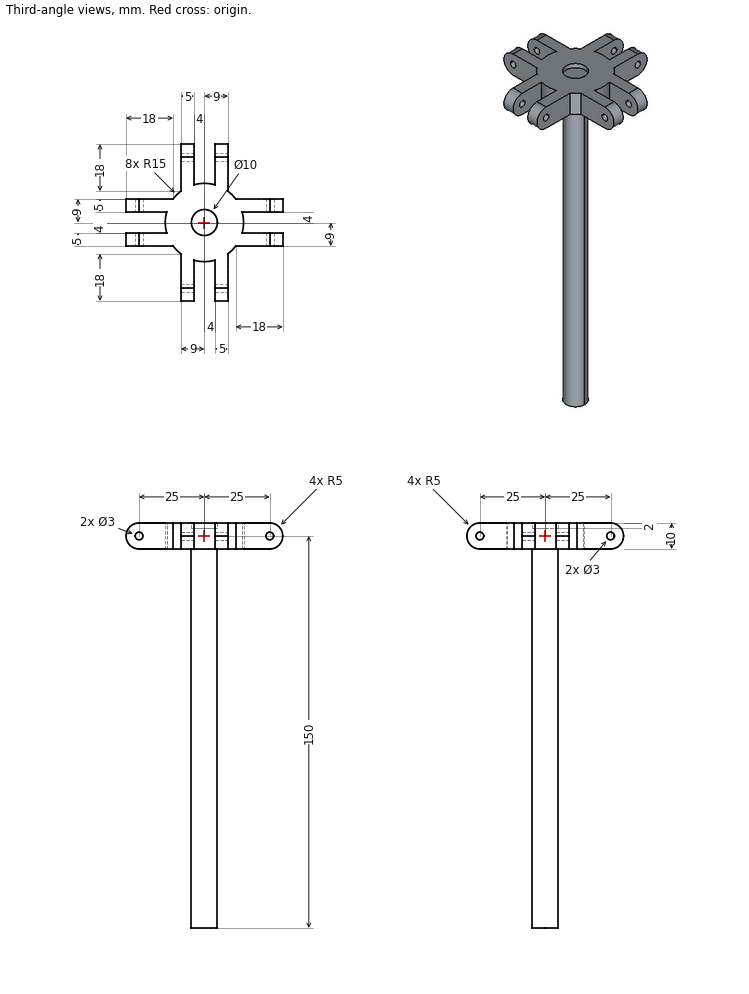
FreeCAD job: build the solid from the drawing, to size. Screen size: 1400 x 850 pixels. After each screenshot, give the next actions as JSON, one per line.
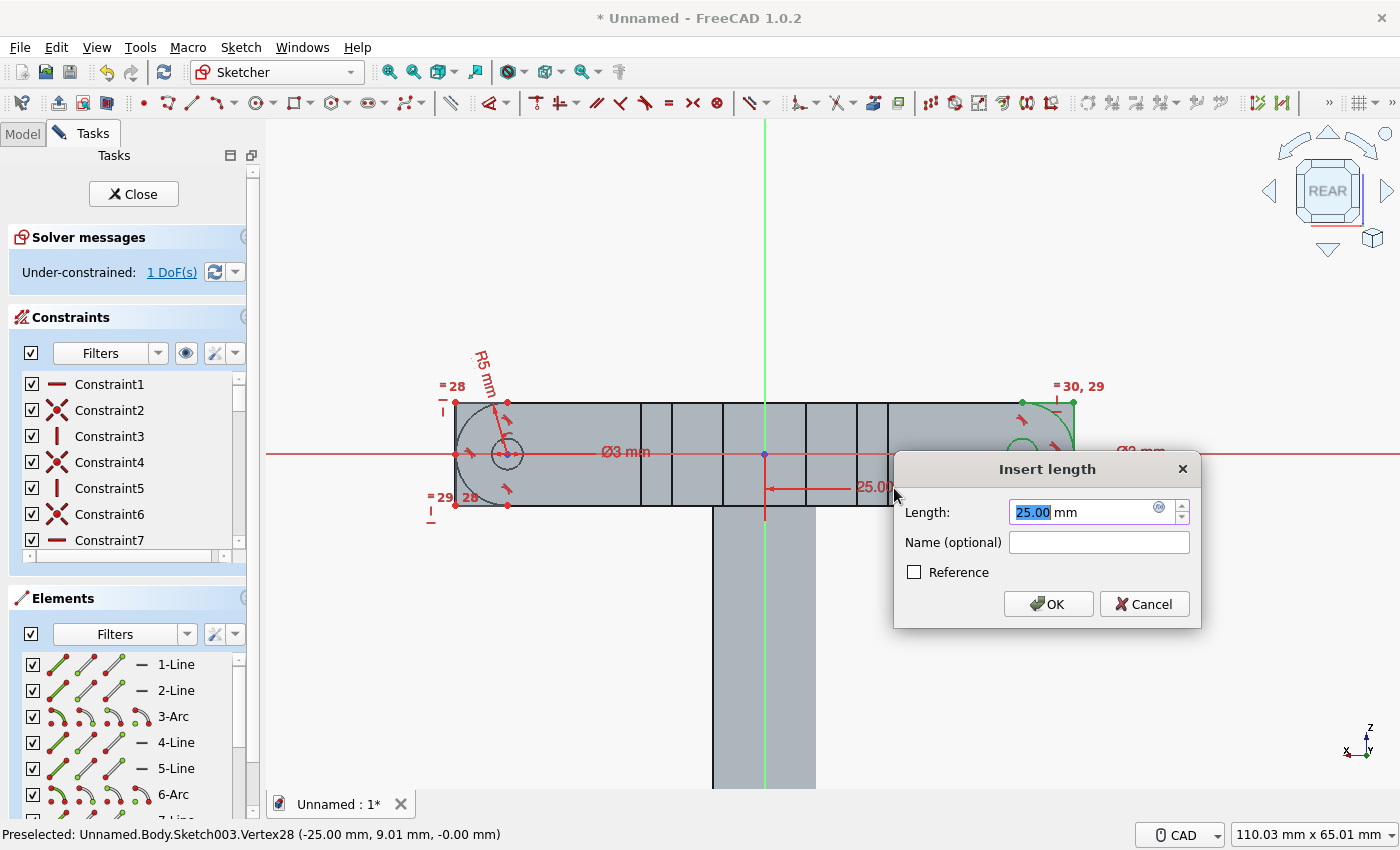
{"action": "type", "text": "25"}
{"action": "key", "text": "Return"}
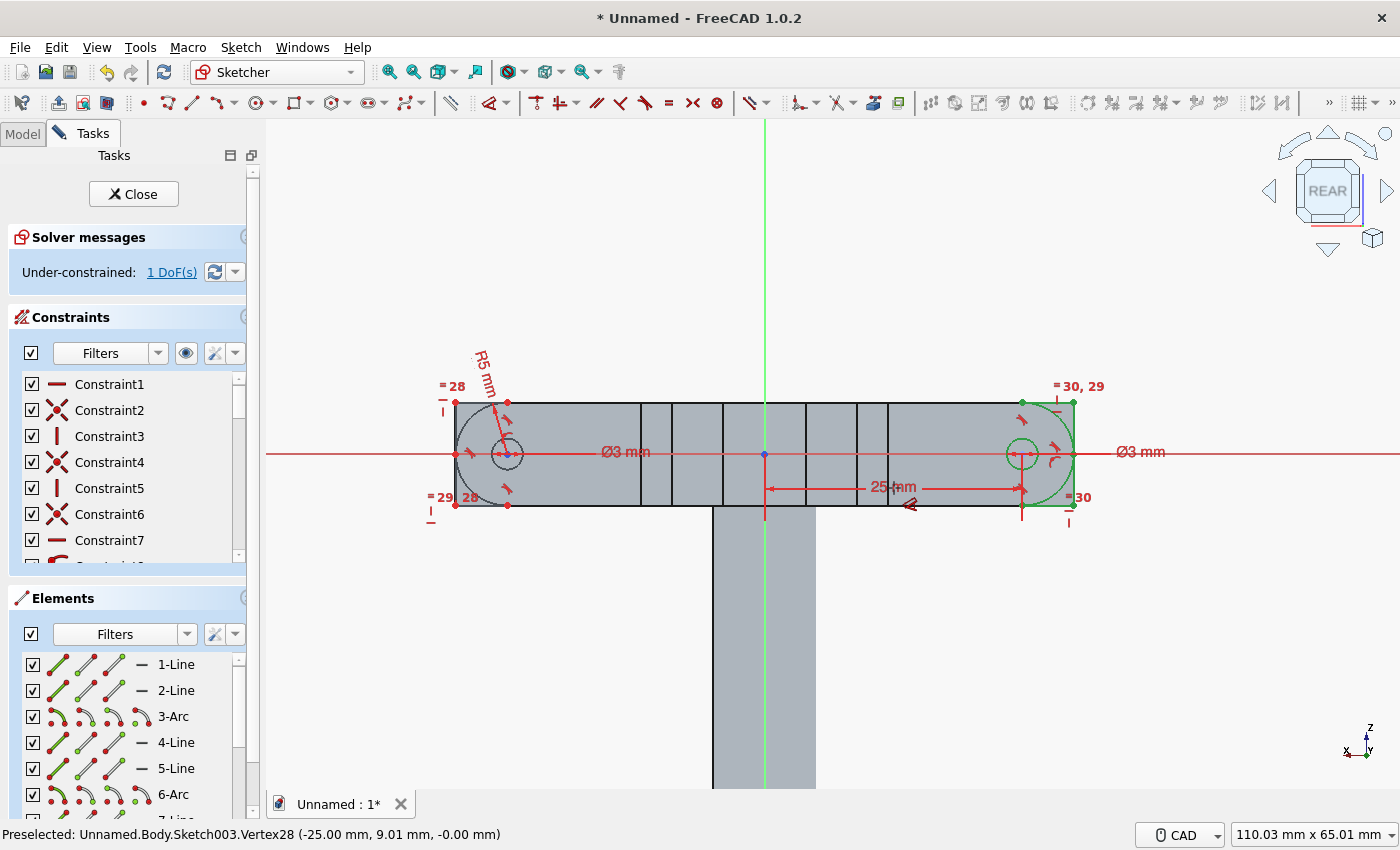
{"action": "left_click", "coordinate": [507, 454]}
{"action": "left_click", "coordinate": [636, 488]}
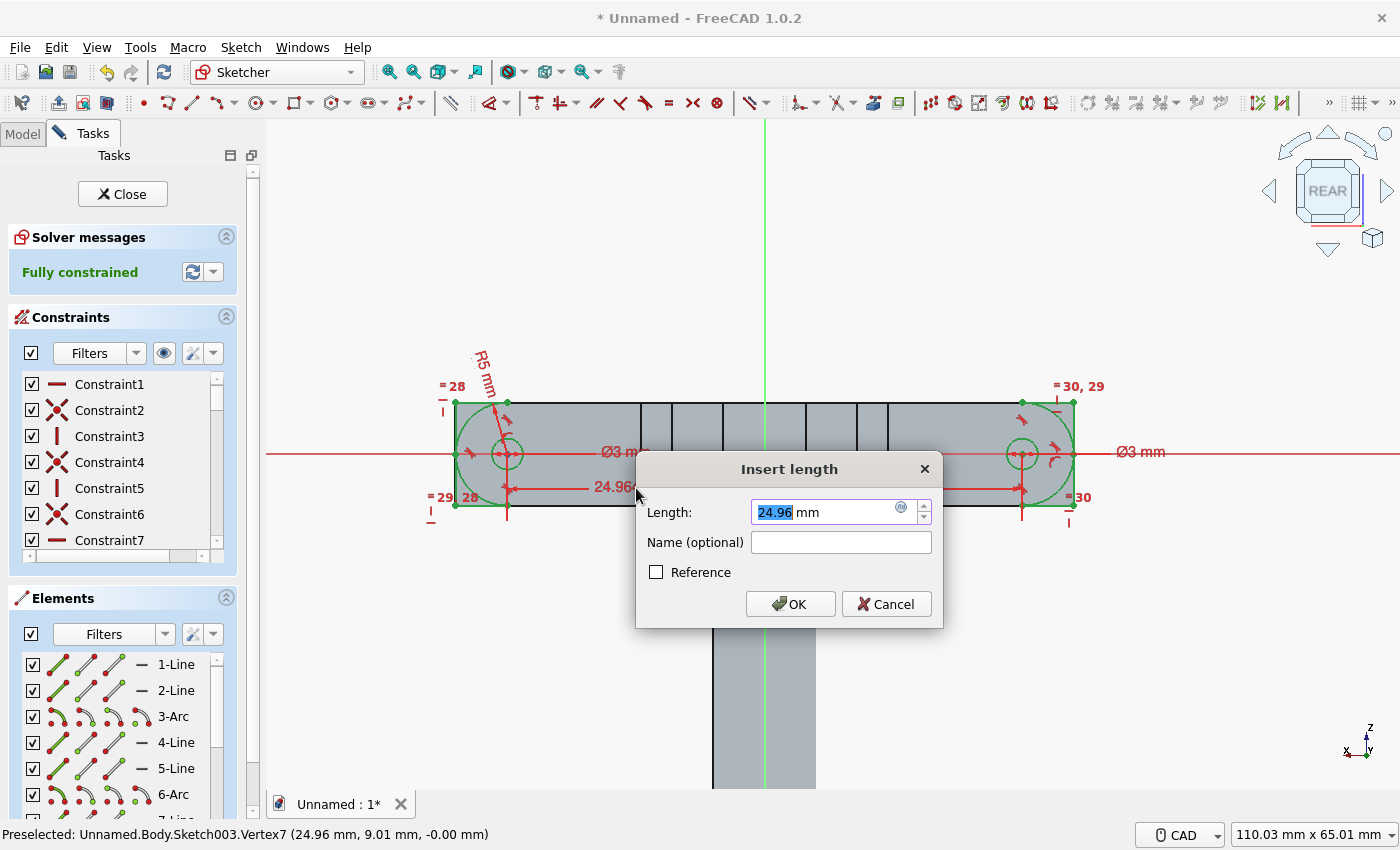
{"action": "type", "text": "25"}
{"action": "key", "text": "Return"}
{"action": "key", "text": "Escape"}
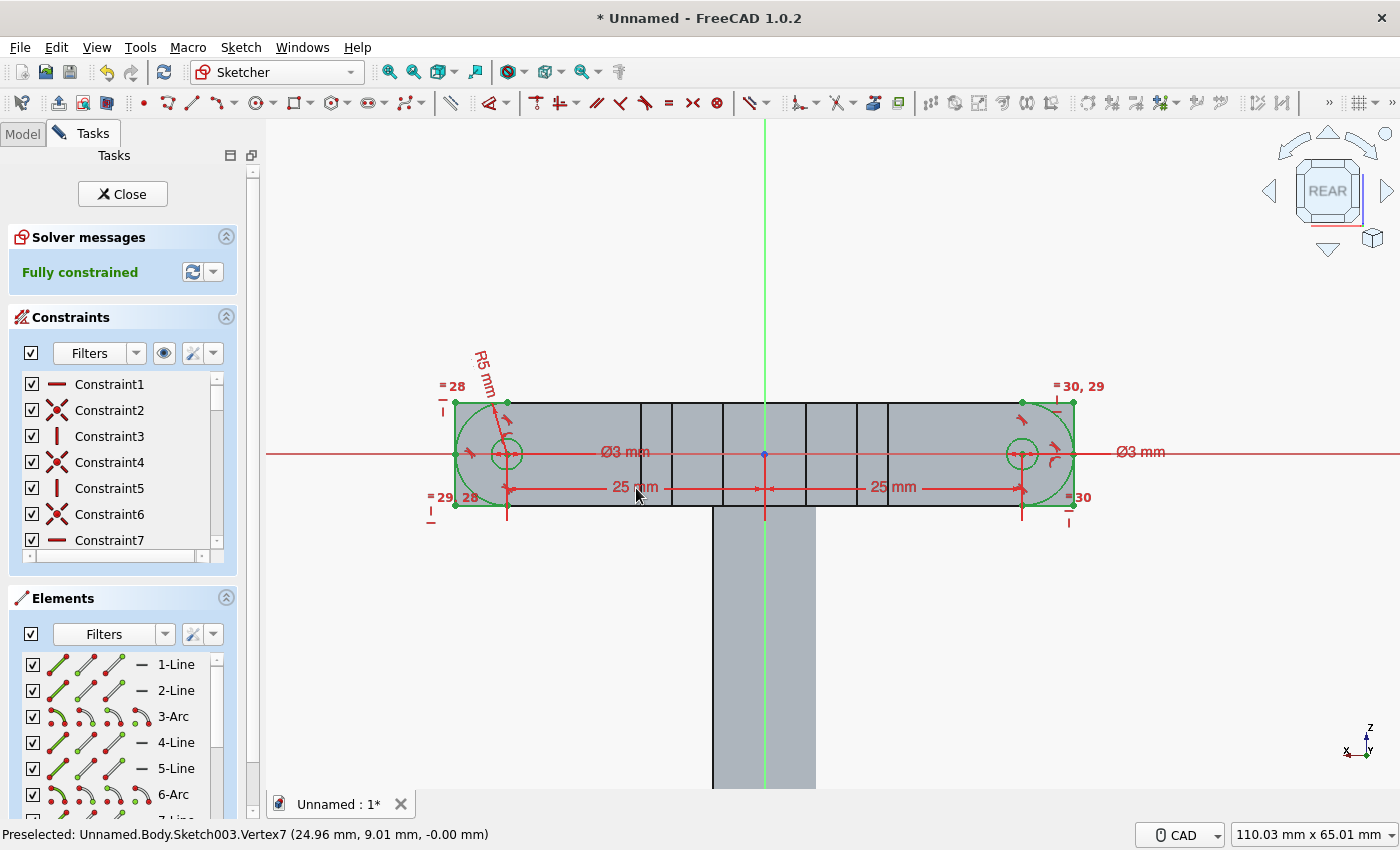
{"action": "left_click", "coordinate": [123, 194]}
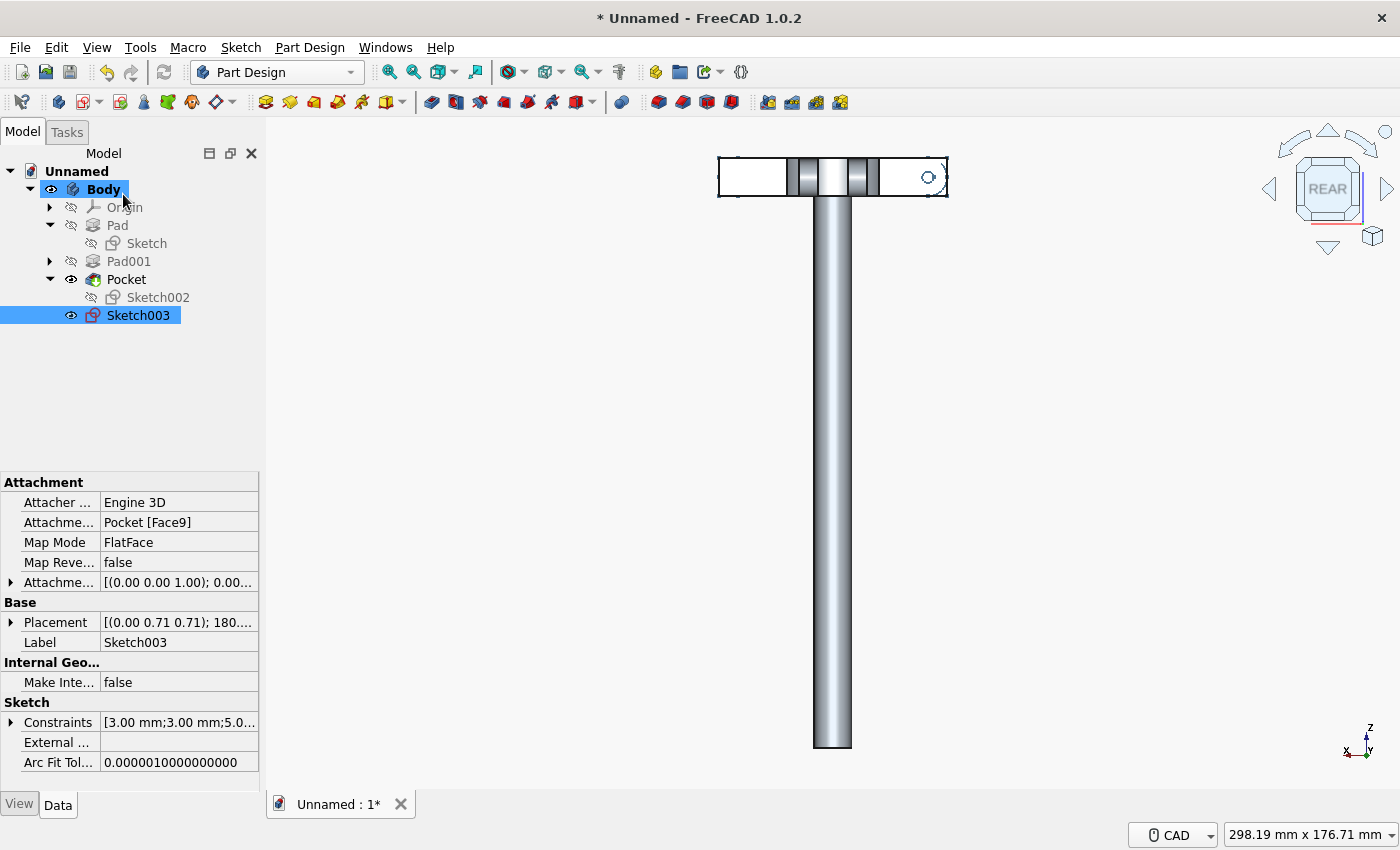
{"action": "left_click", "coordinate": [432, 102]}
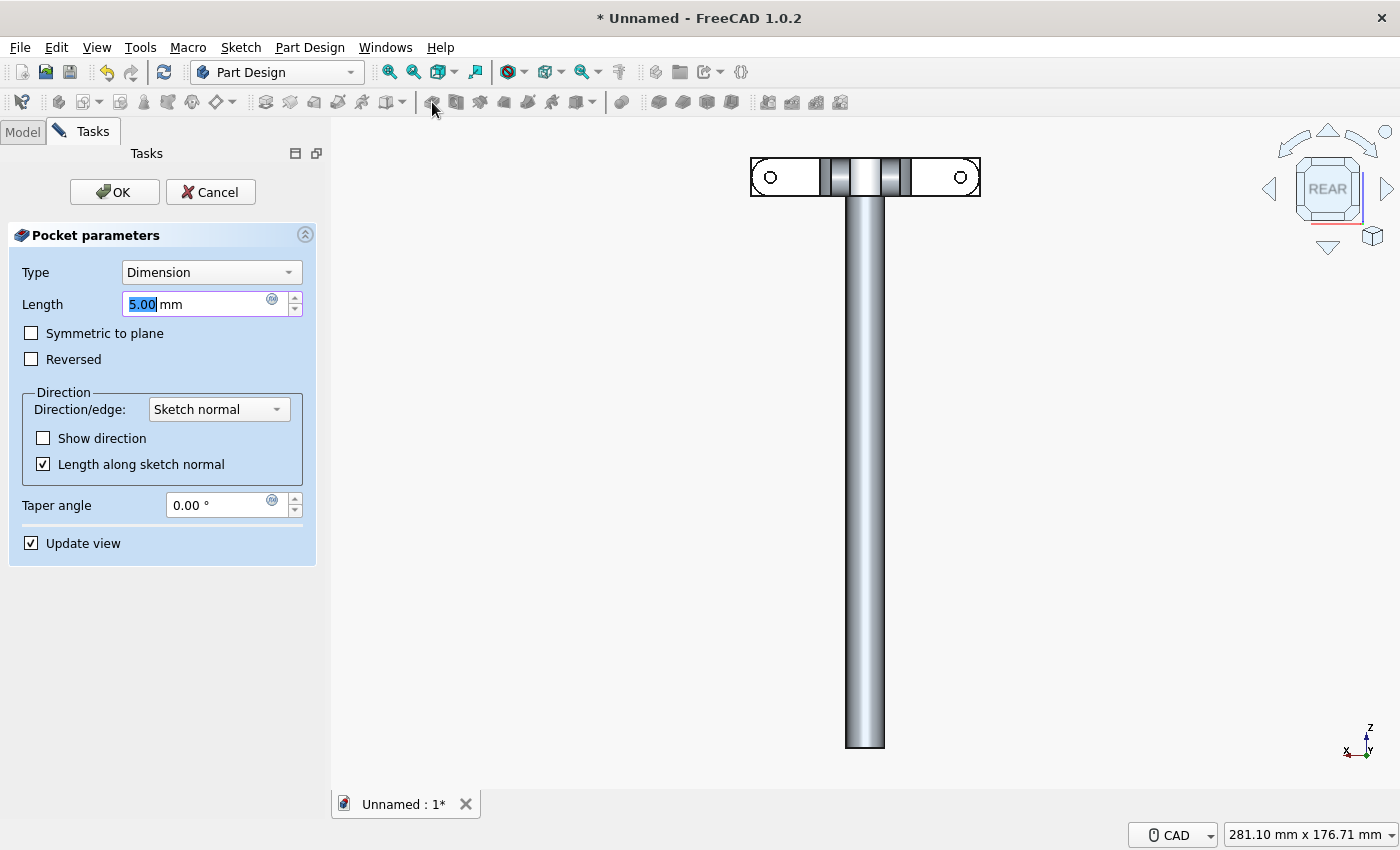
{"action": "left_click", "coordinate": [212, 272]}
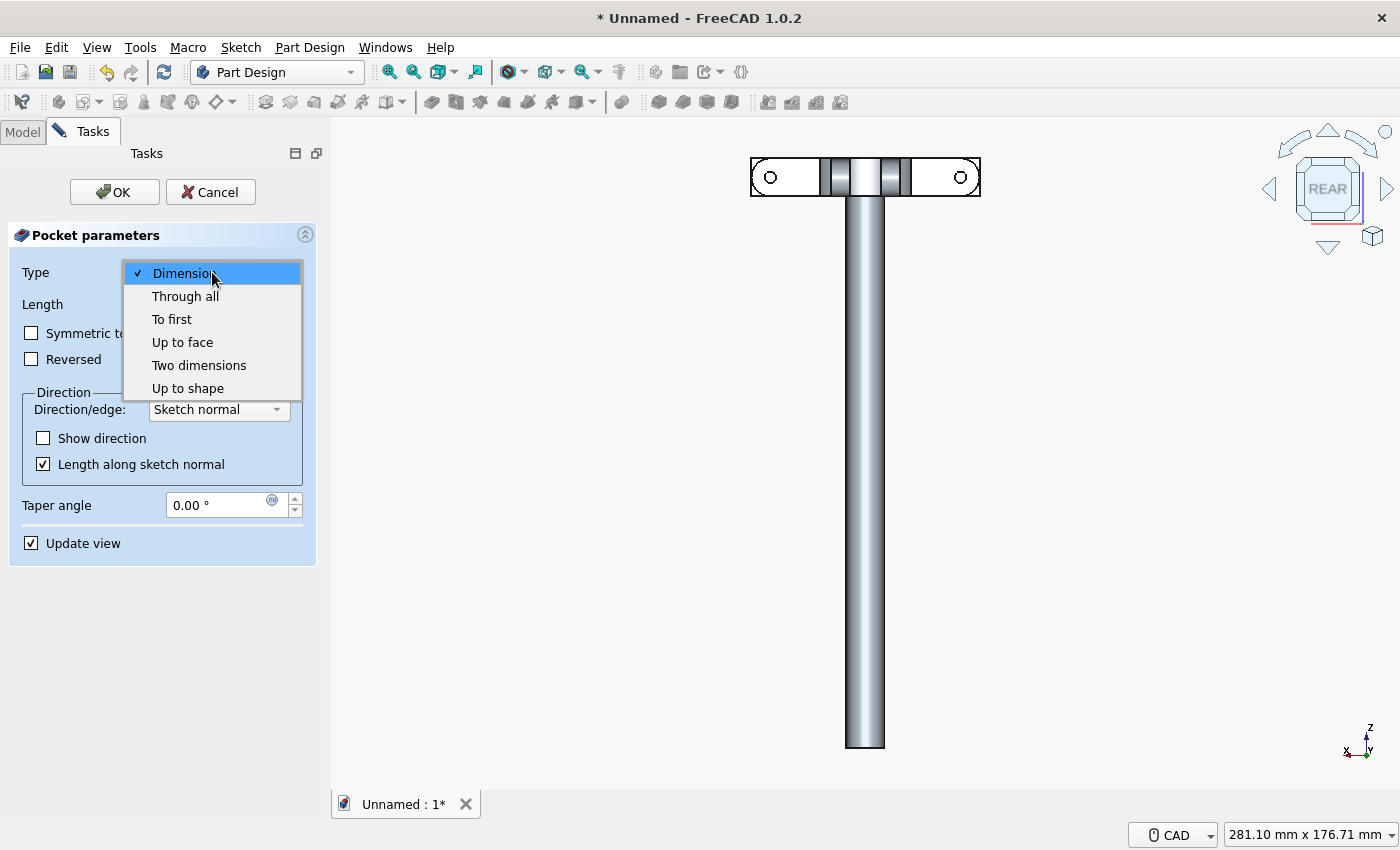
{"action": "left_click", "coordinate": [212, 296]}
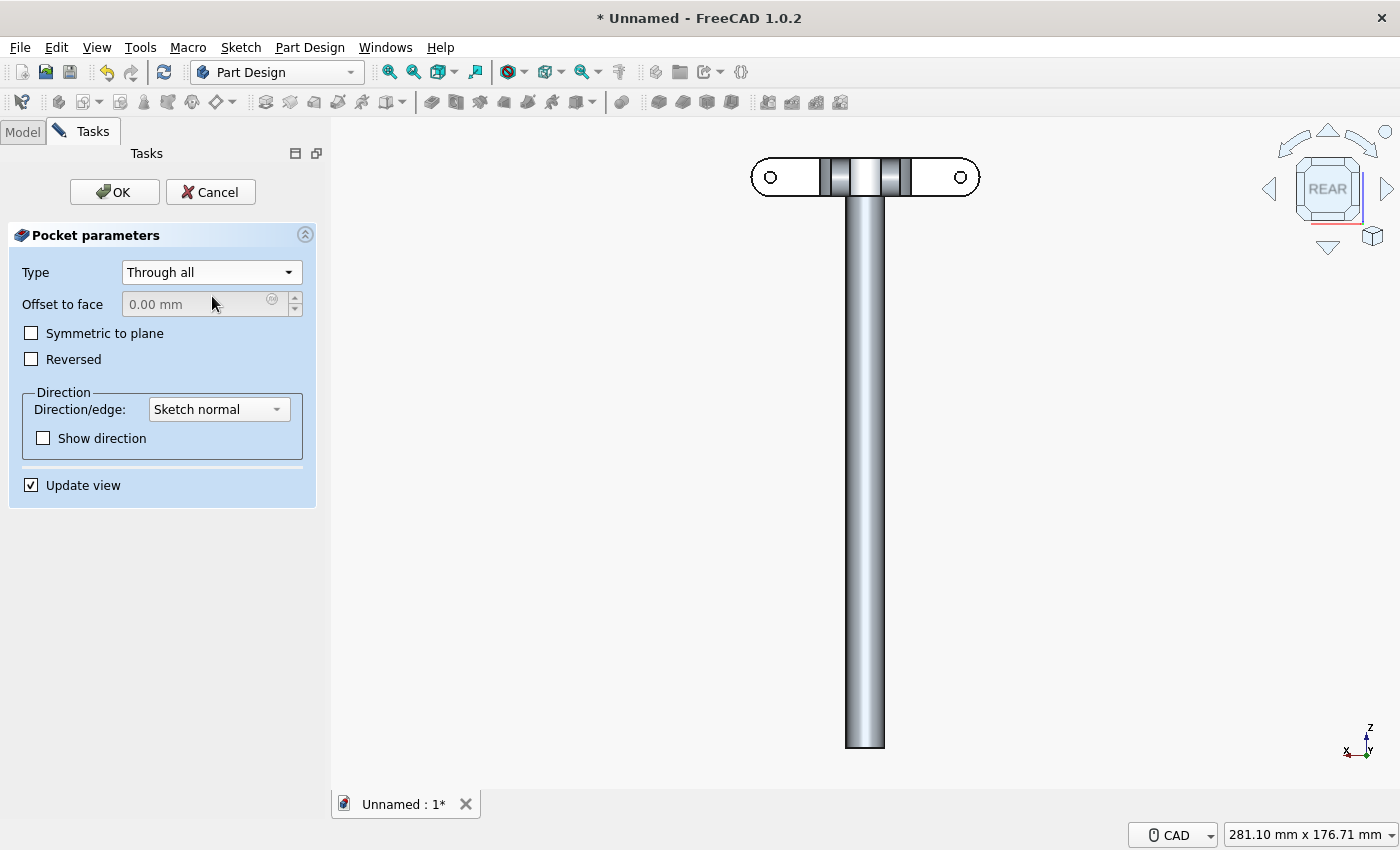
{"action": "left_click", "coordinate": [115, 192]}